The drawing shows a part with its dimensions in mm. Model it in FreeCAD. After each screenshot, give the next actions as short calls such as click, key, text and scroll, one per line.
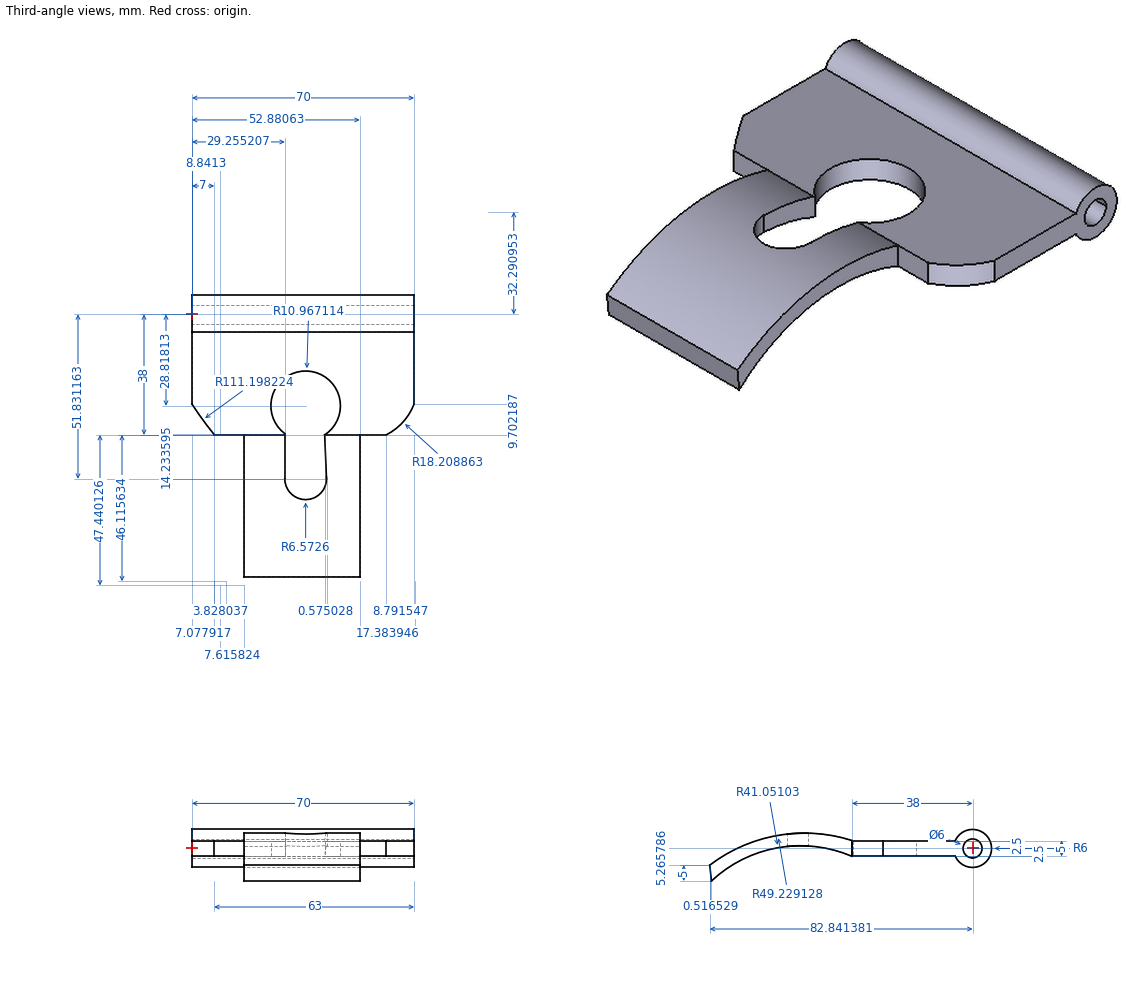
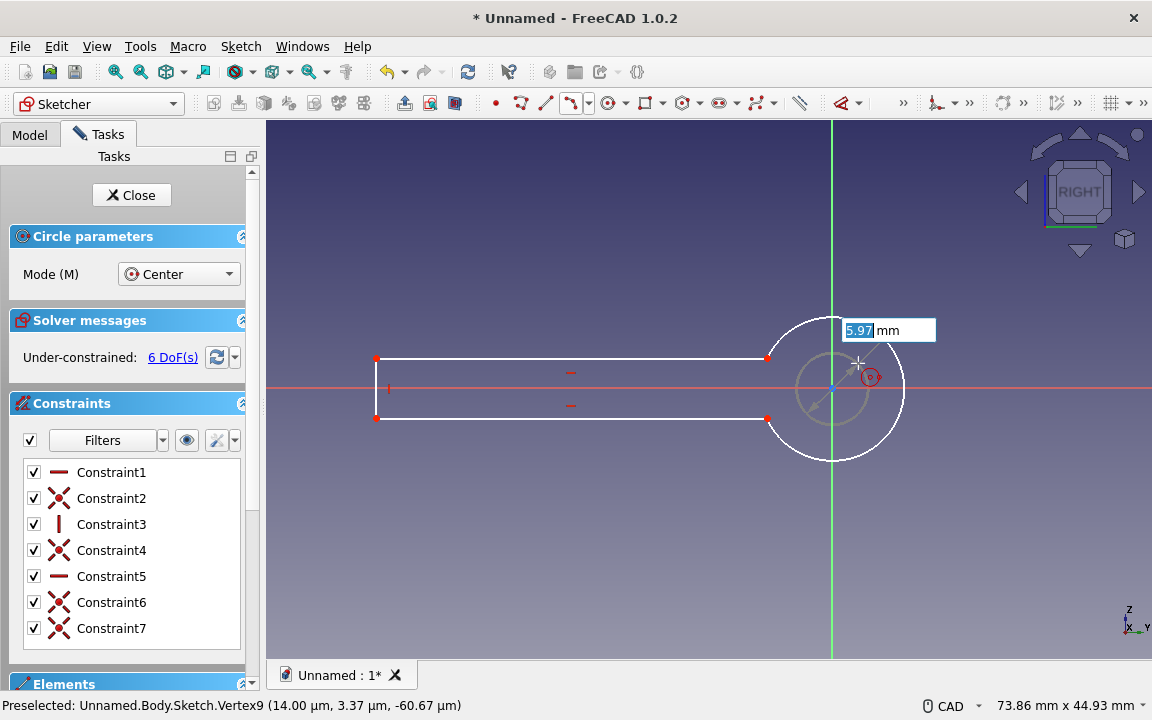
text(6)
key(Return)
key(Escape)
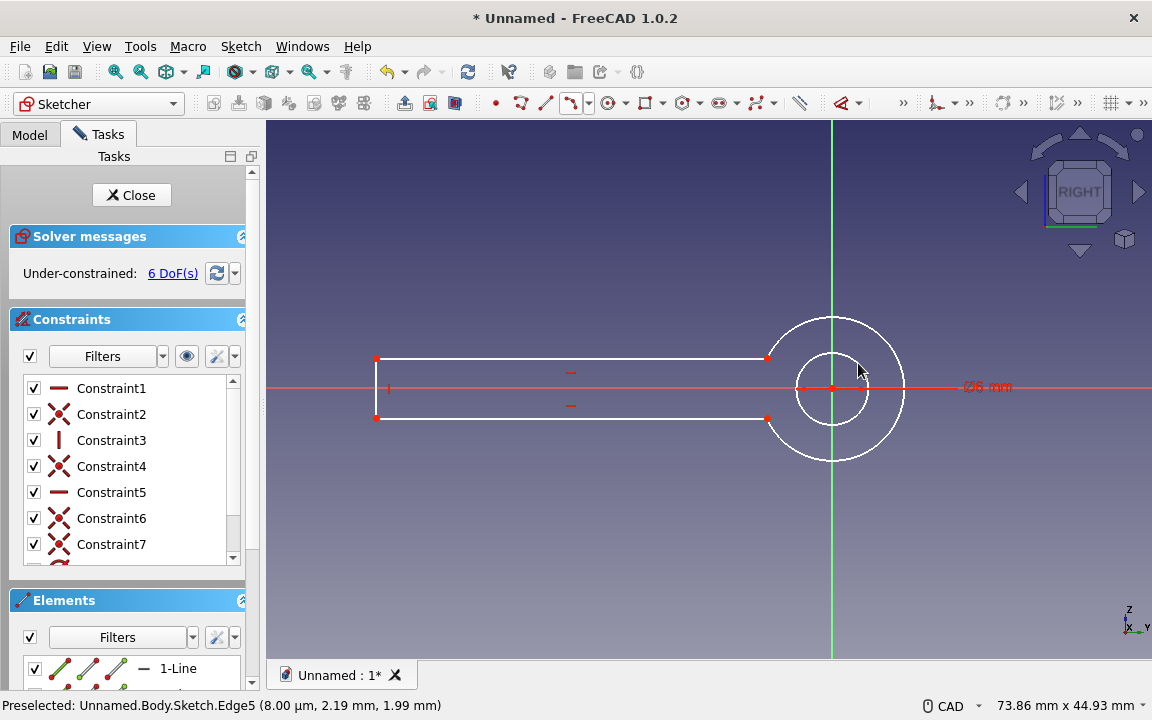
drag(822, 378, 842, 399)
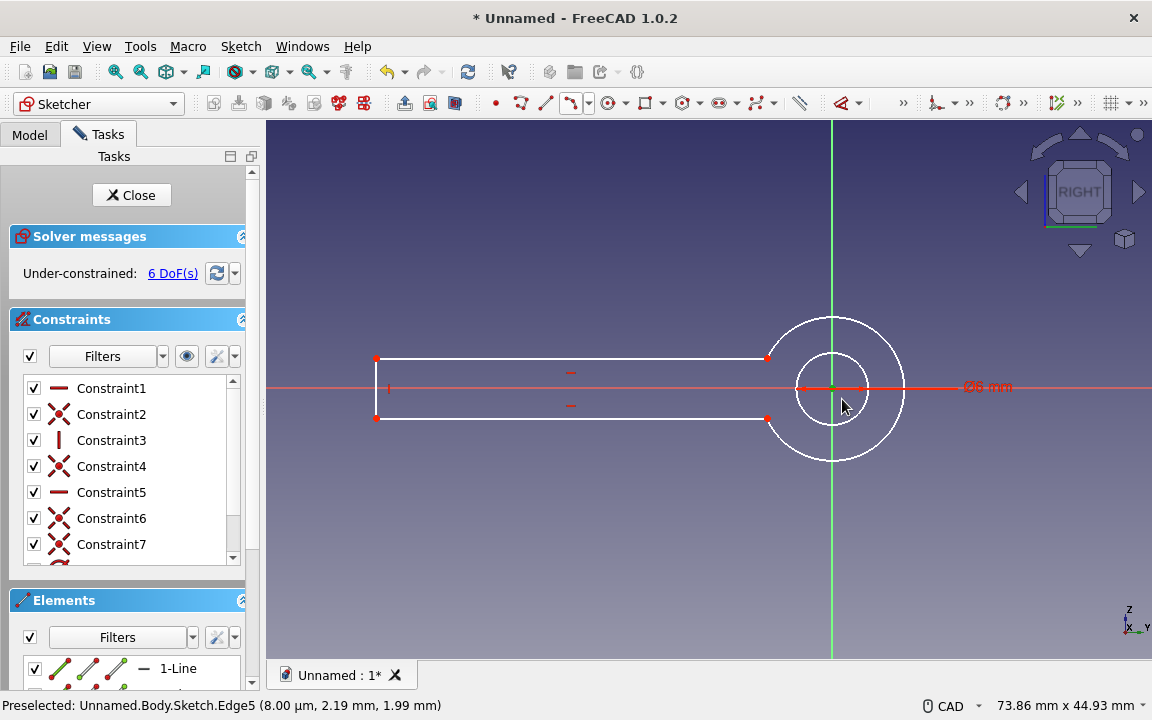
key(c)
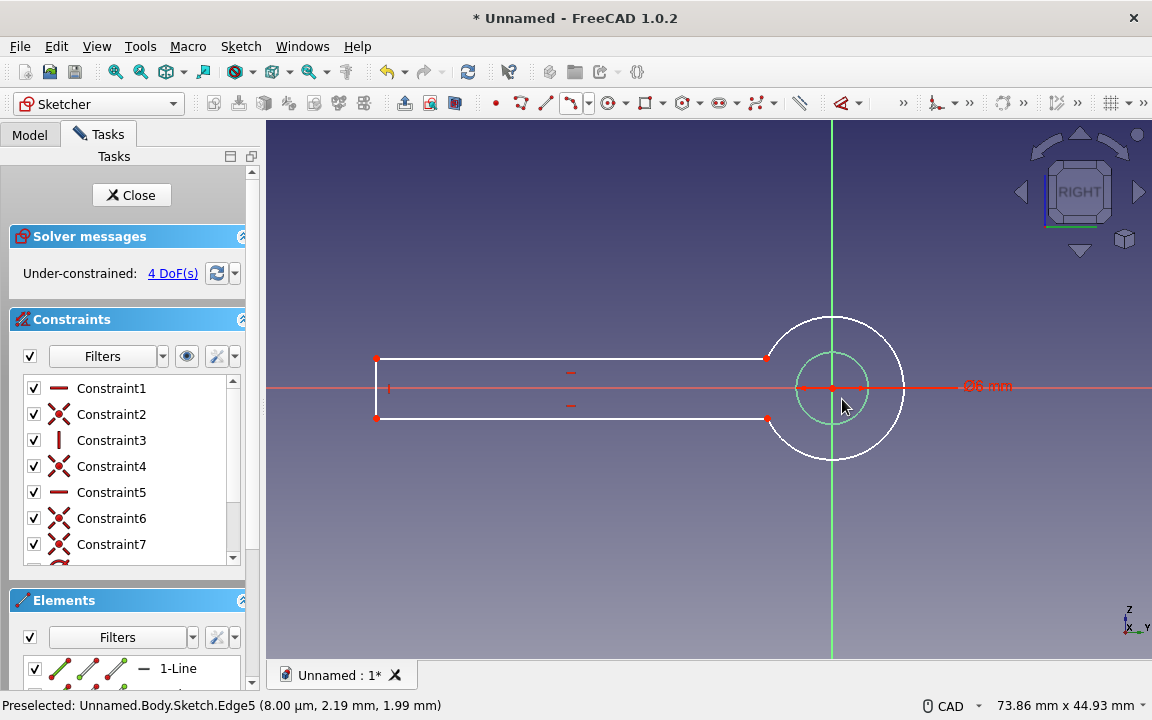
click(867, 451)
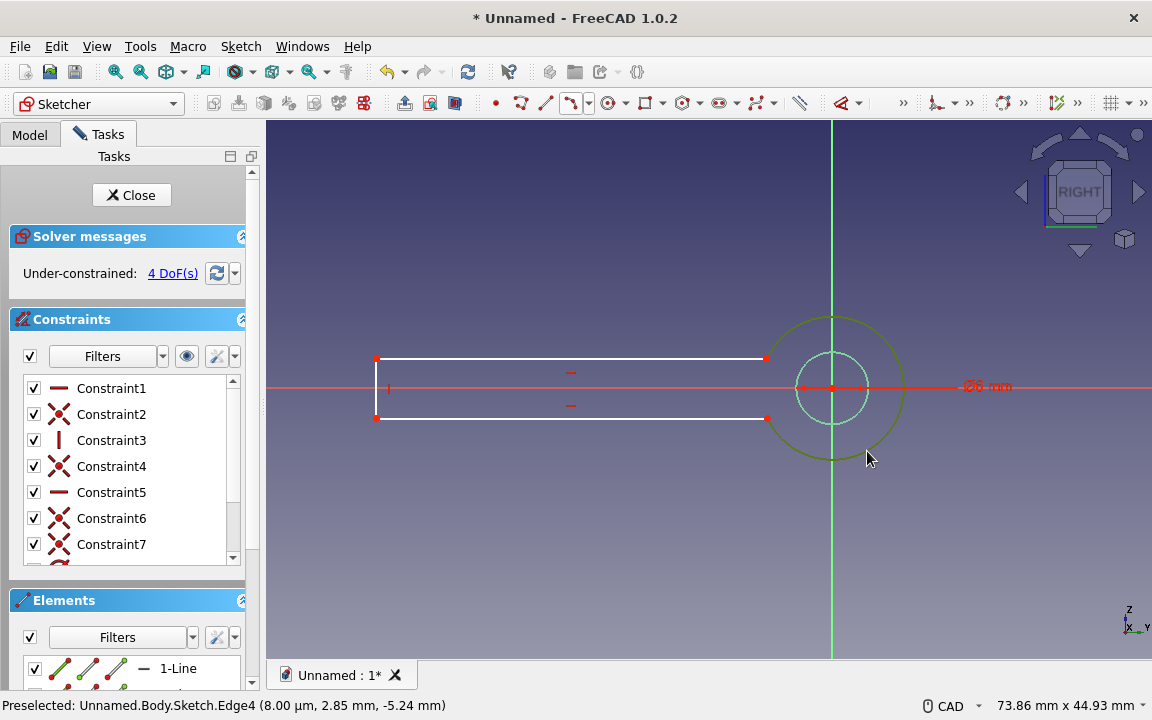
key(k)
key(r)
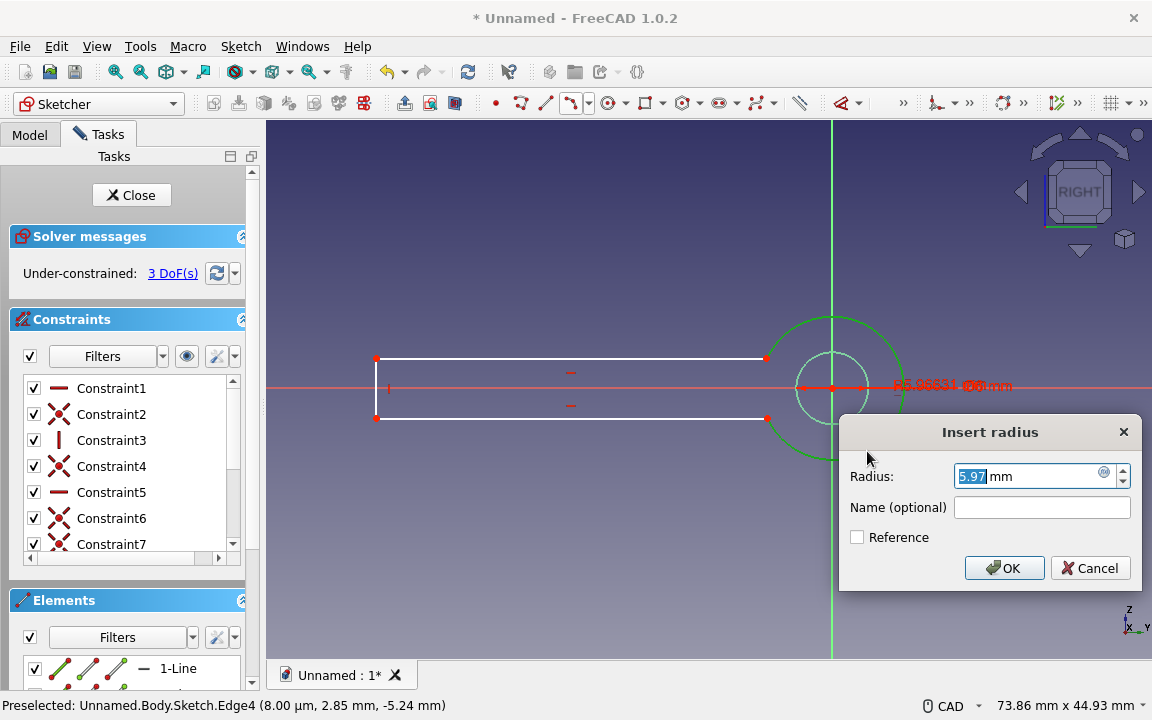
text(6)
key(Return)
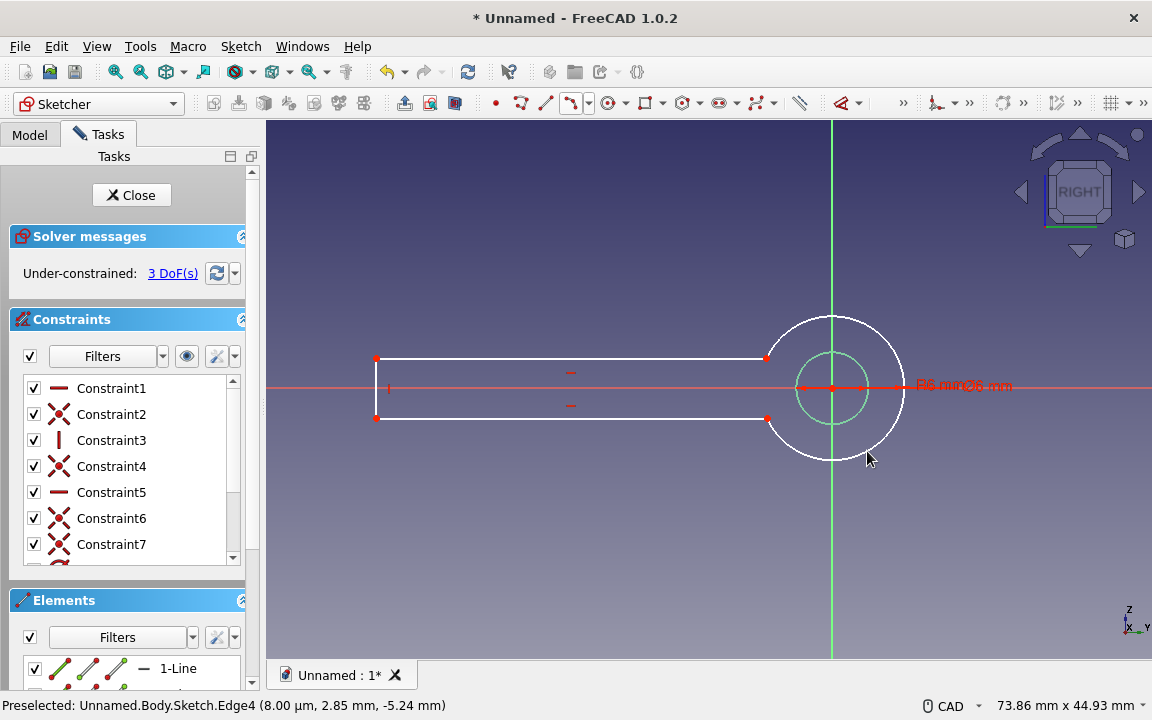
scroll(376, 377, up, 2)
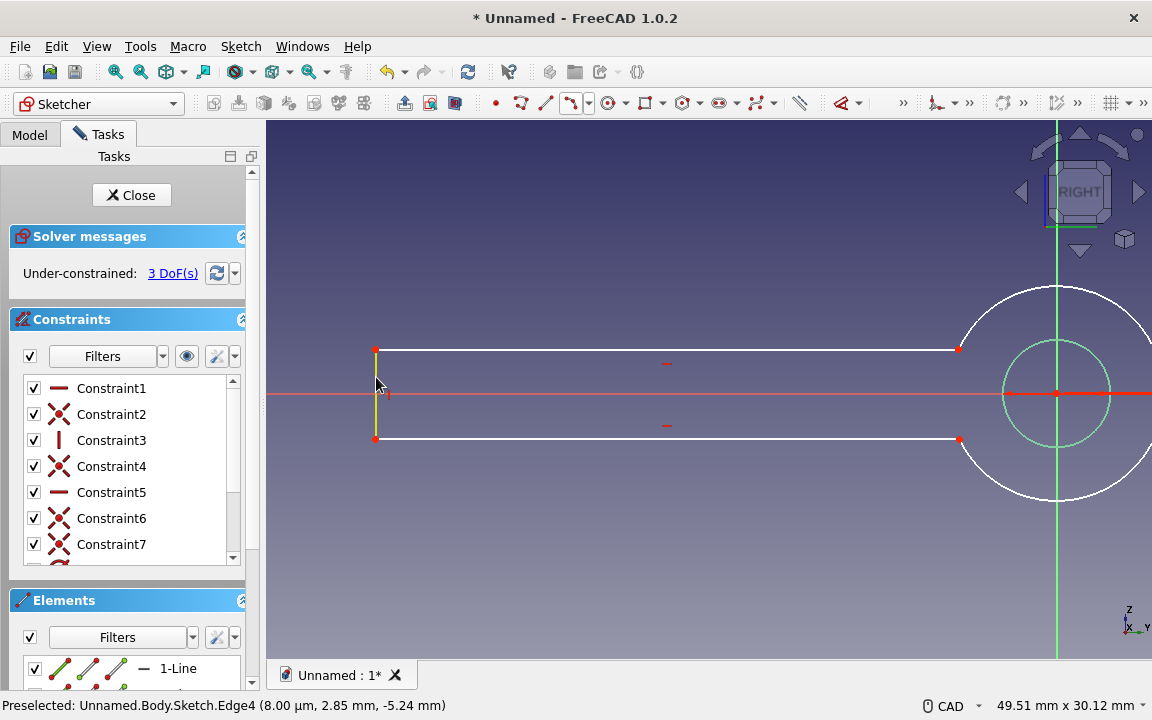
click(376, 377)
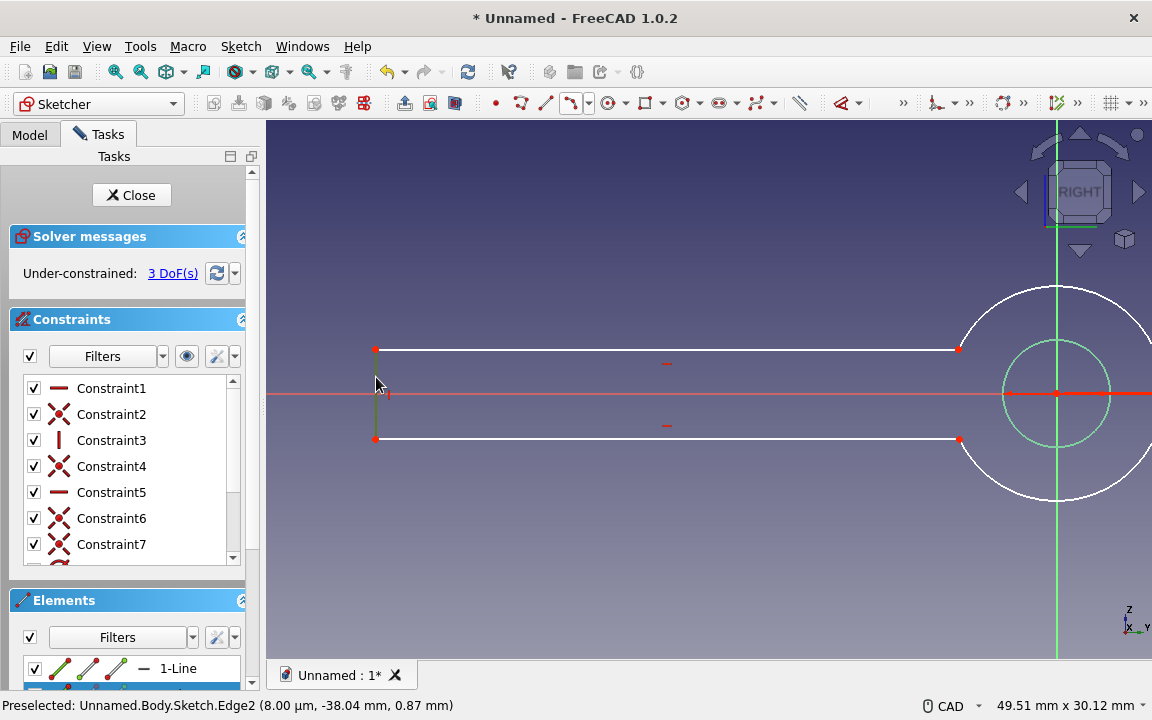
key(i)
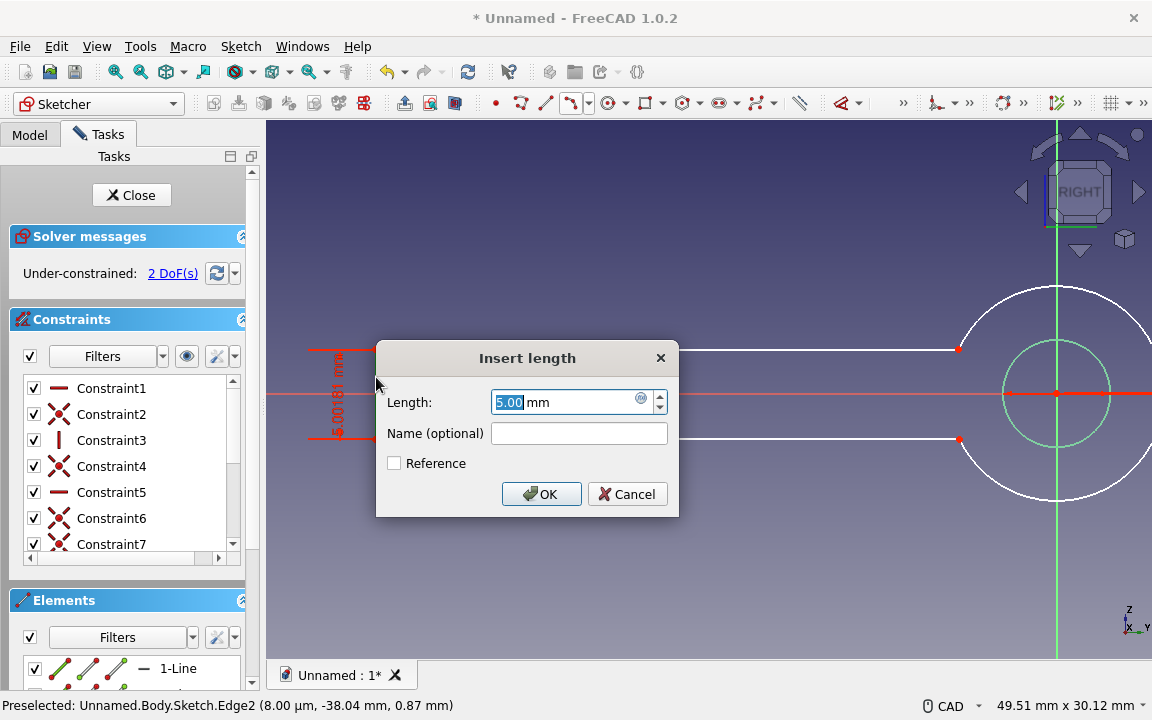
text(5)
key(Return)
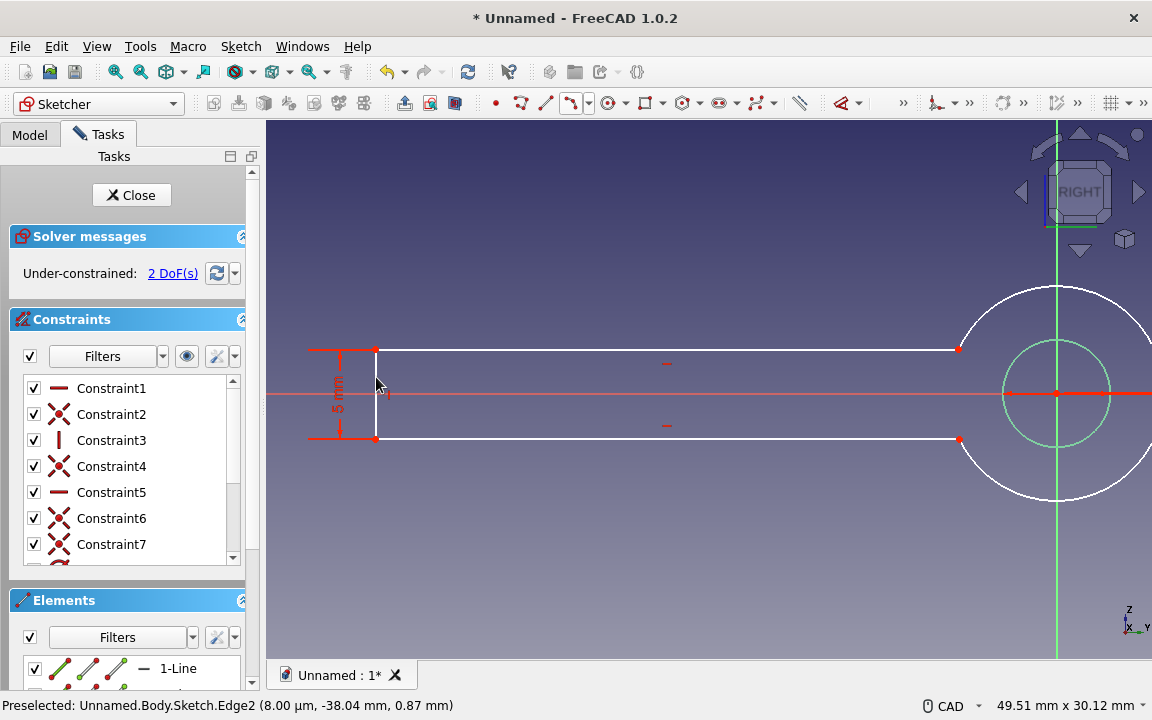
click(376, 350)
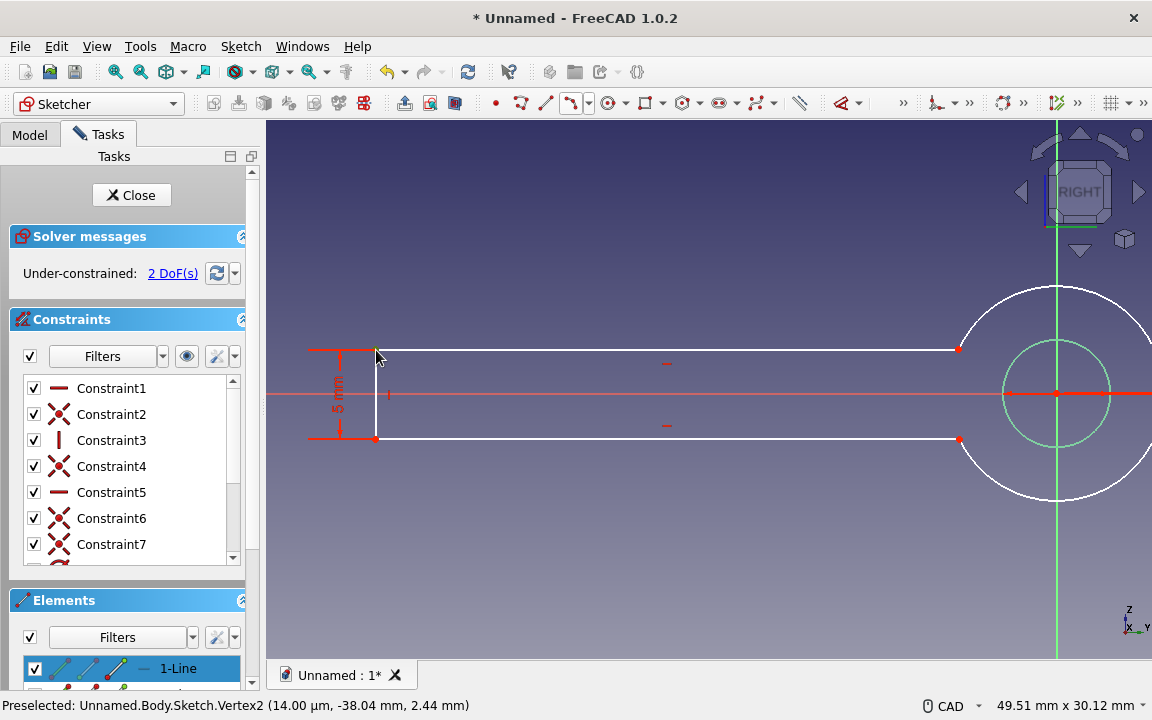
key(l)